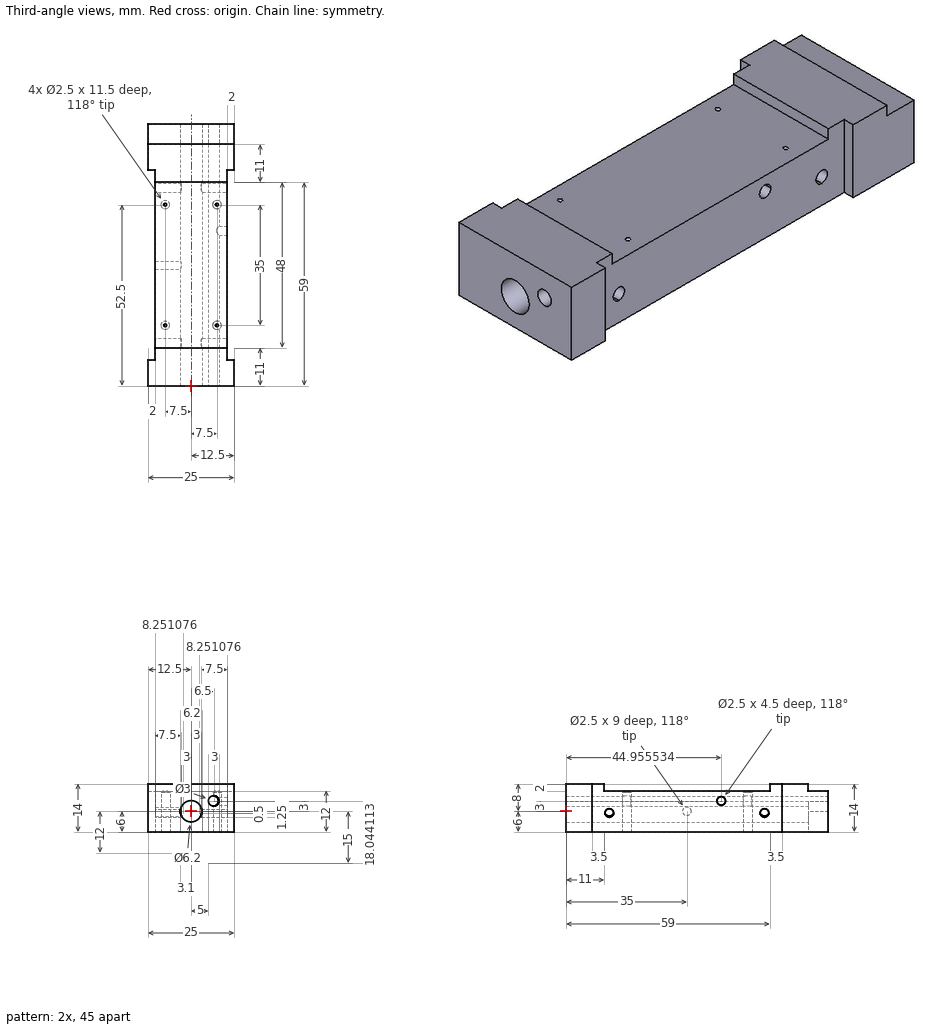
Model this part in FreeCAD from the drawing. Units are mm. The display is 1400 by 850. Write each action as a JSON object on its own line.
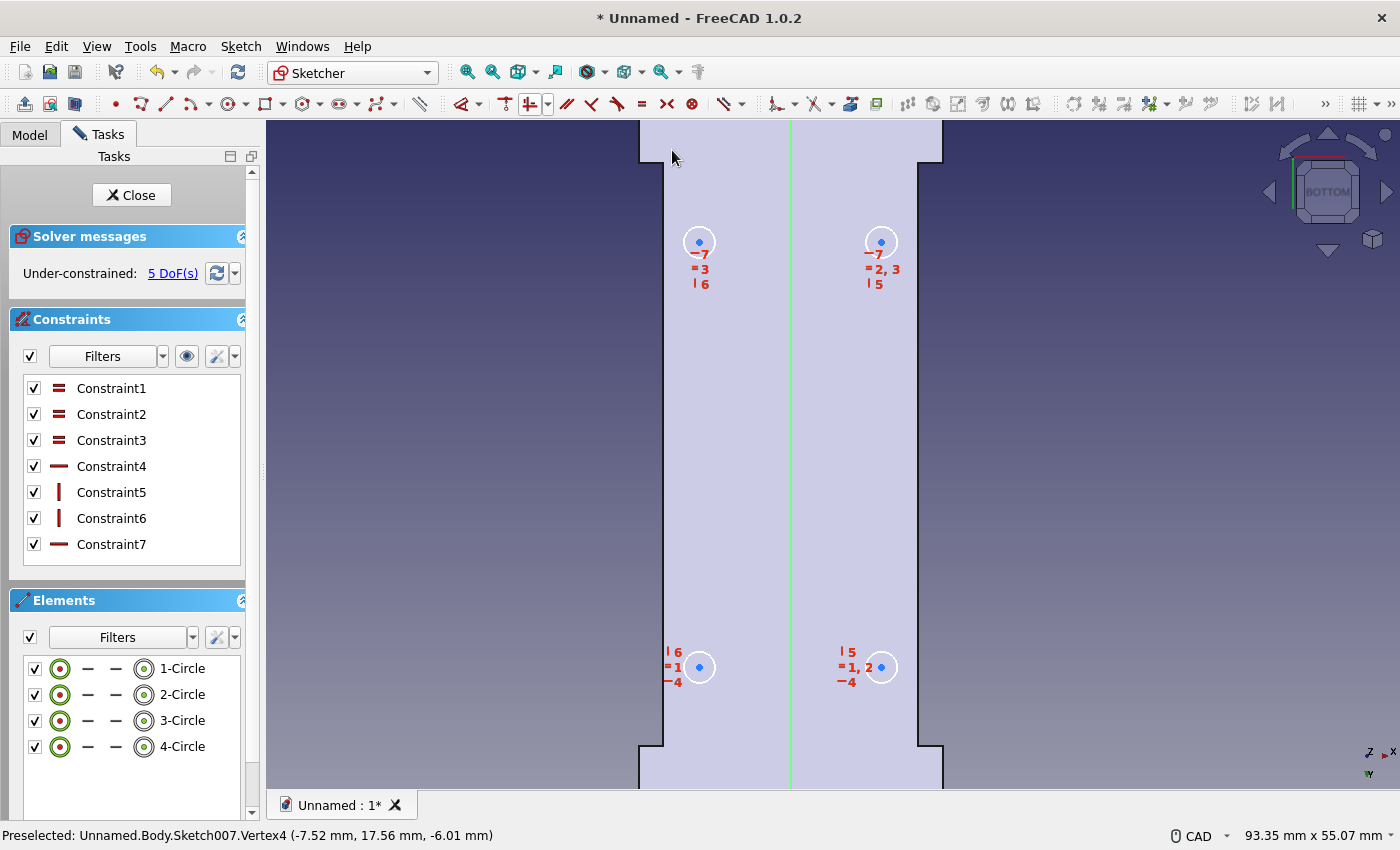
{"action": "left_click", "coordinate": [460, 104]}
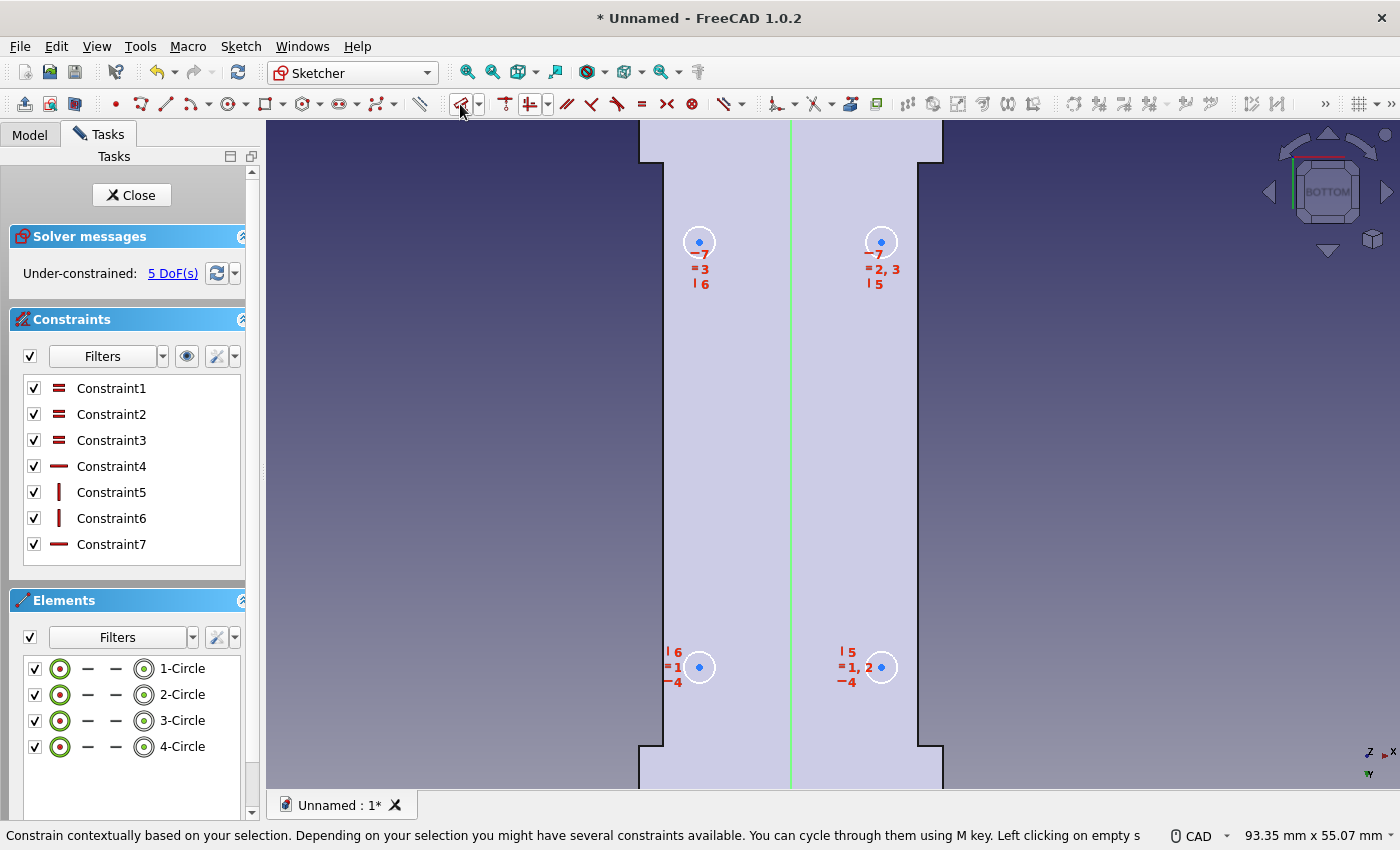
{"action": "scroll", "coordinate": [710, 656], "scroll_direction": "up", "scroll_amount": 2}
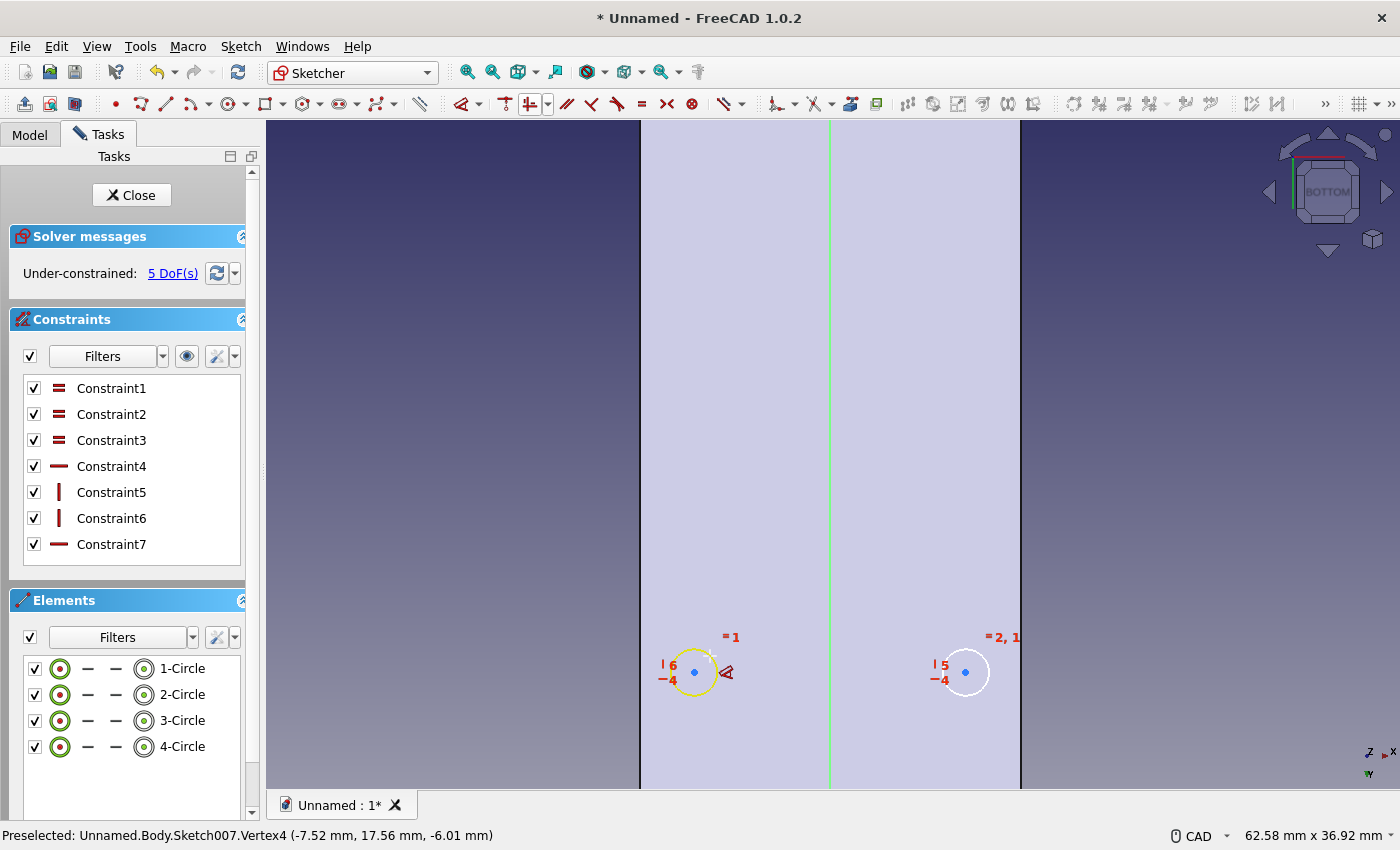
{"action": "left_click", "coordinate": [710, 656]}
{"action": "left_click", "coordinate": [732, 633]}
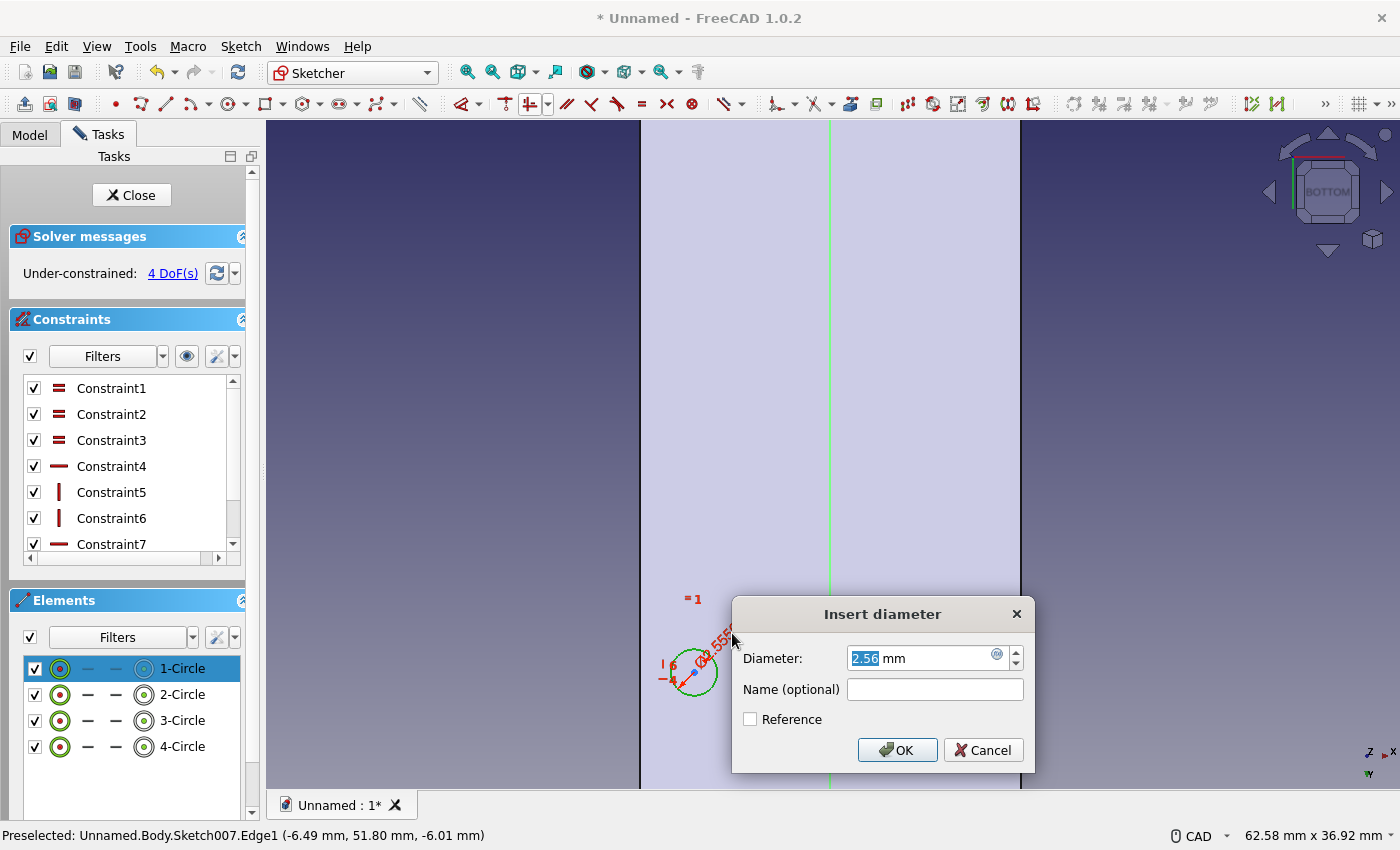
{"action": "type", "text": "2.5"}
{"action": "key", "text": "Return"}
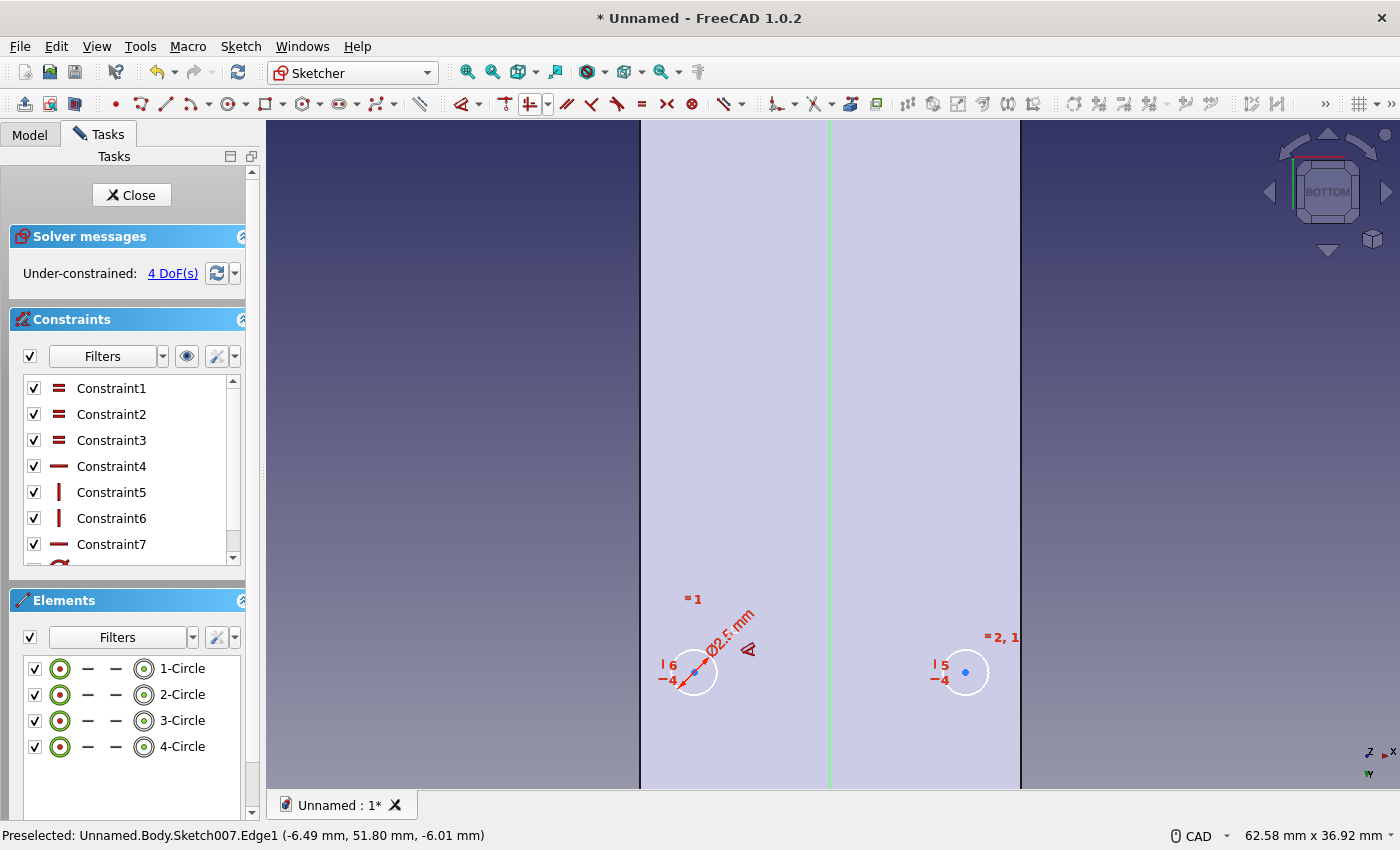
{"action": "left_click", "coordinate": [694, 673]}
{"action": "left_click", "coordinate": [762, 707]}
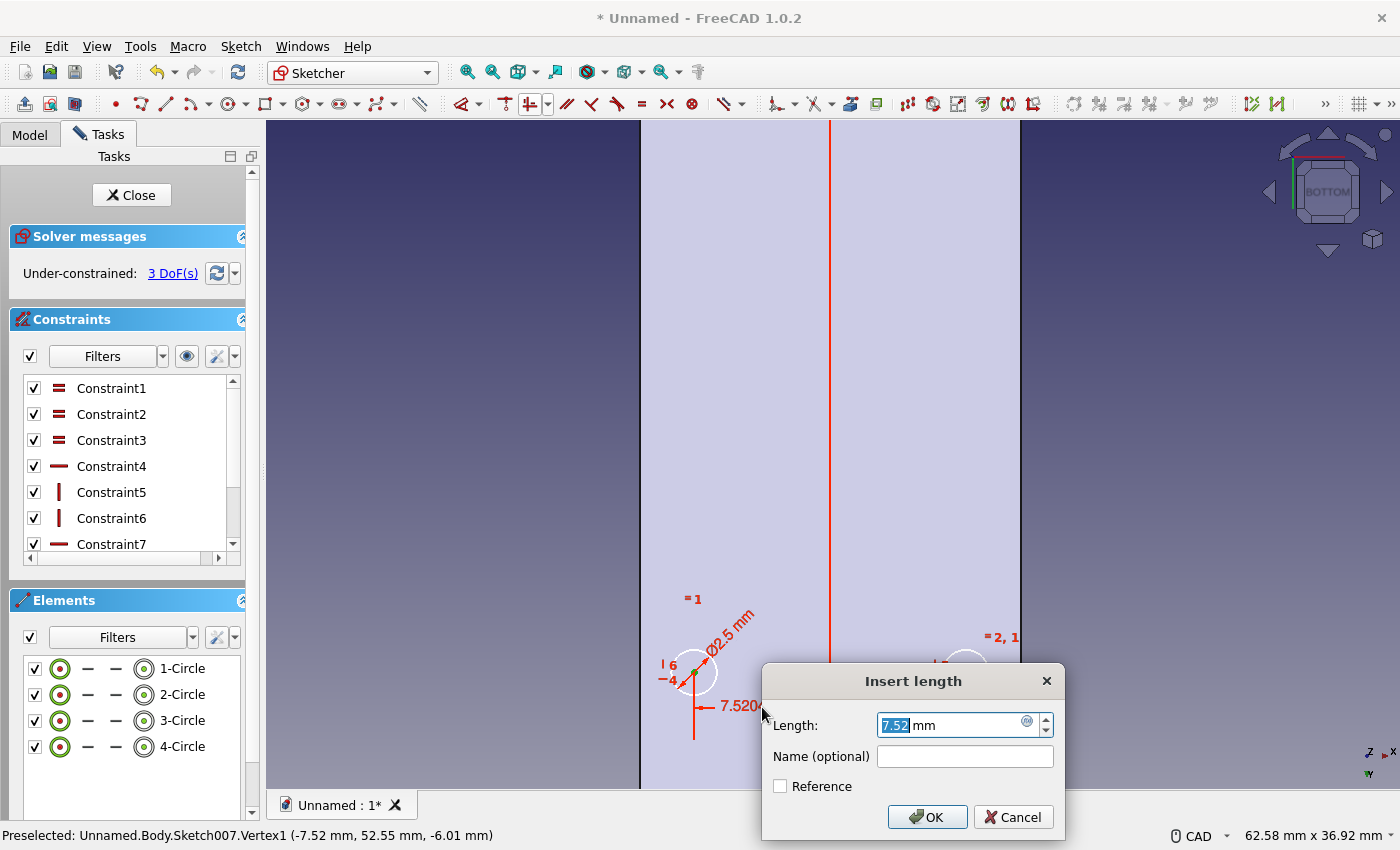
{"action": "type", "text": "7.5"}
{"action": "key", "text": "Return"}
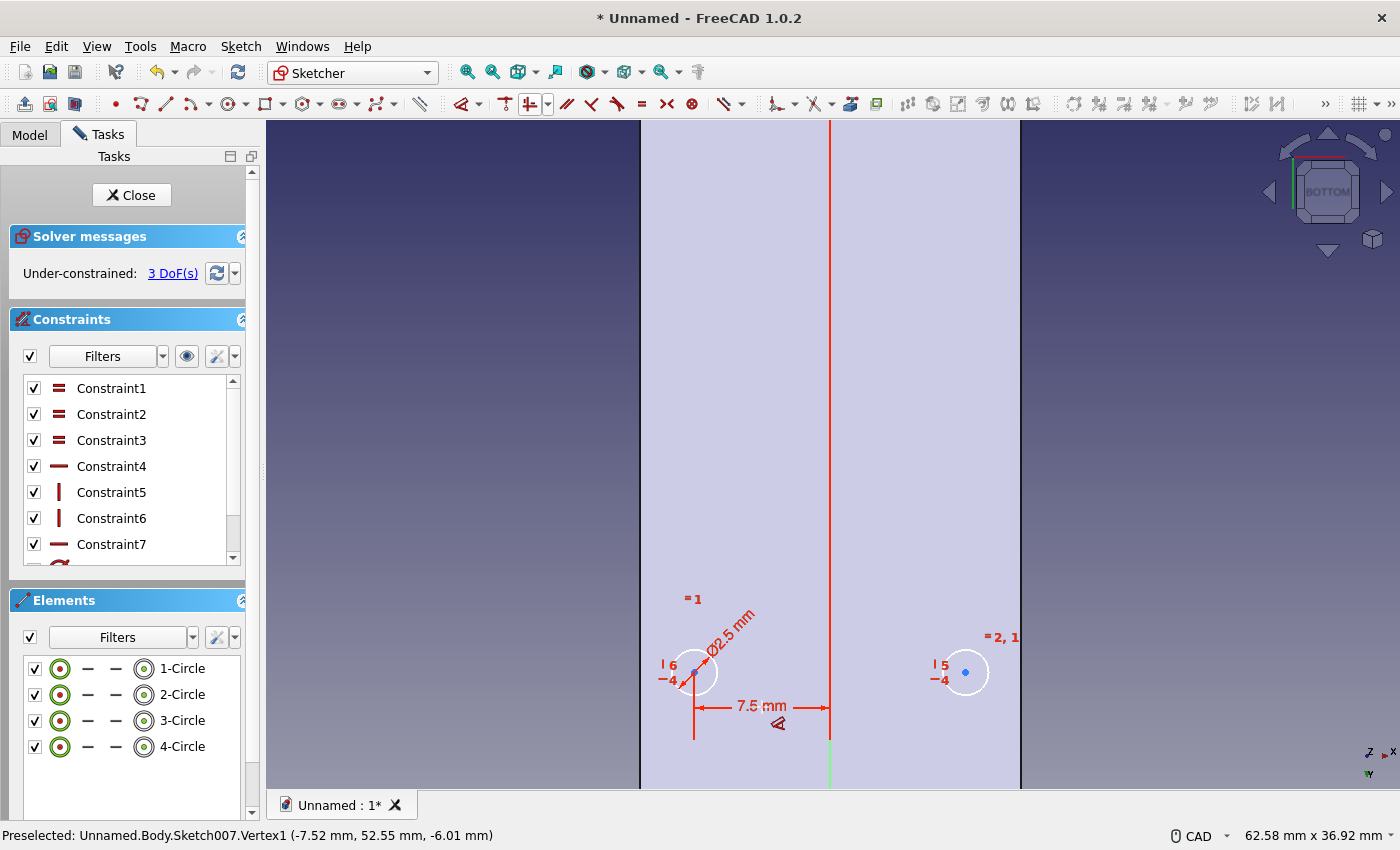
{"action": "left_click", "coordinate": [966, 673]}
{"action": "left_click", "coordinate": [898, 707]}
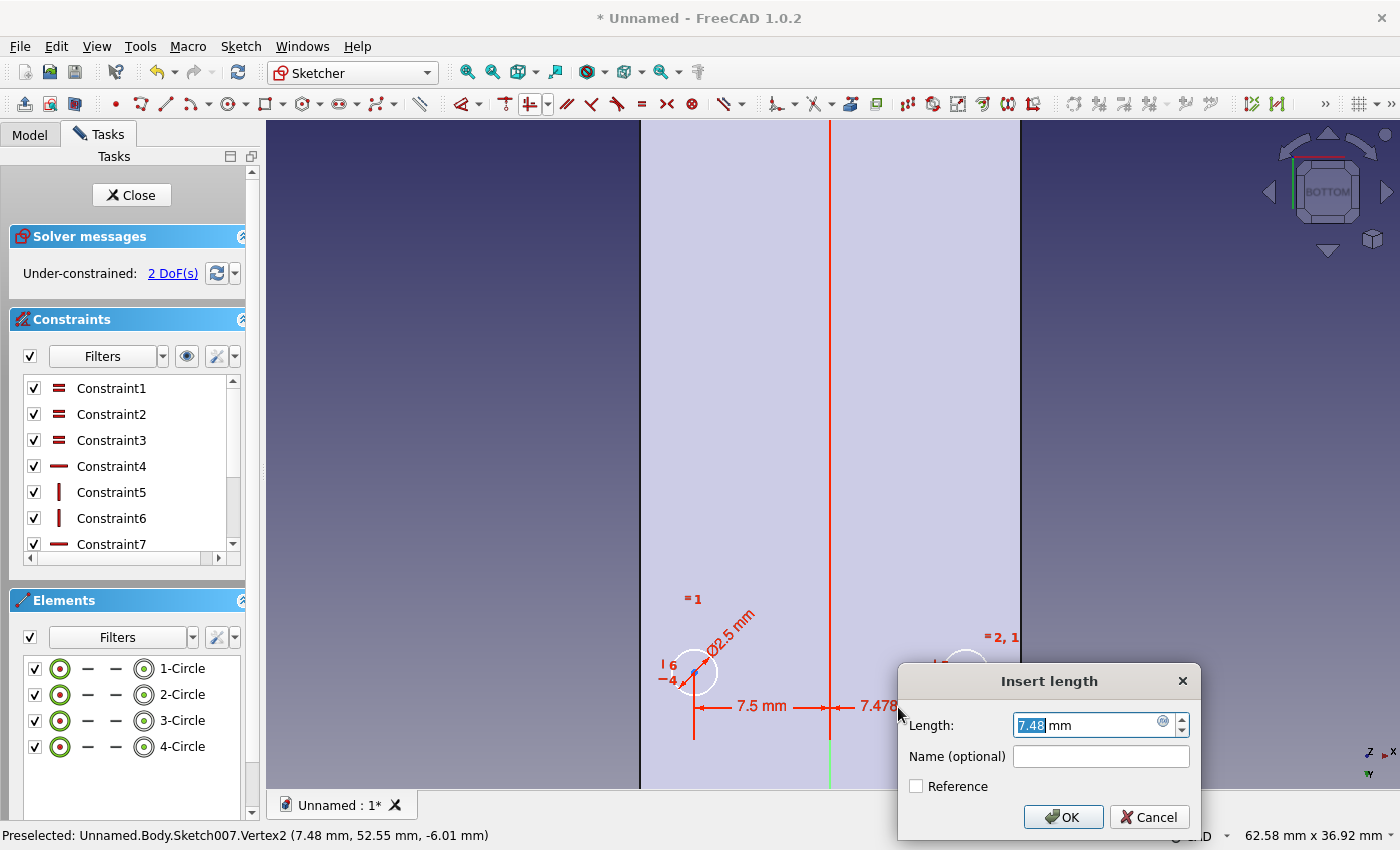
{"action": "type", "text": "7.5"}
{"action": "key", "text": "Return"}